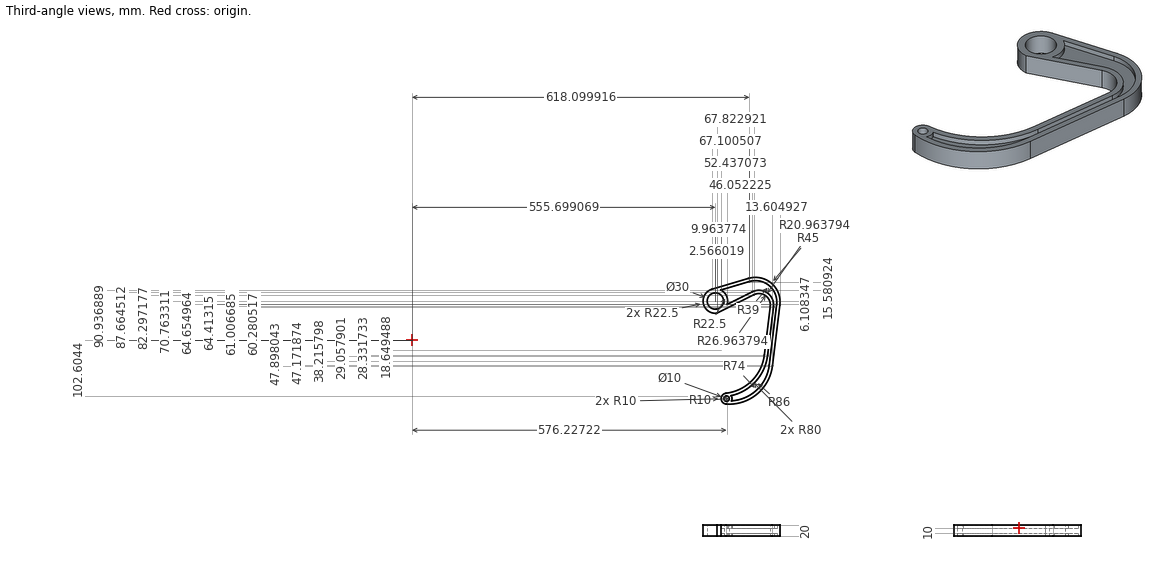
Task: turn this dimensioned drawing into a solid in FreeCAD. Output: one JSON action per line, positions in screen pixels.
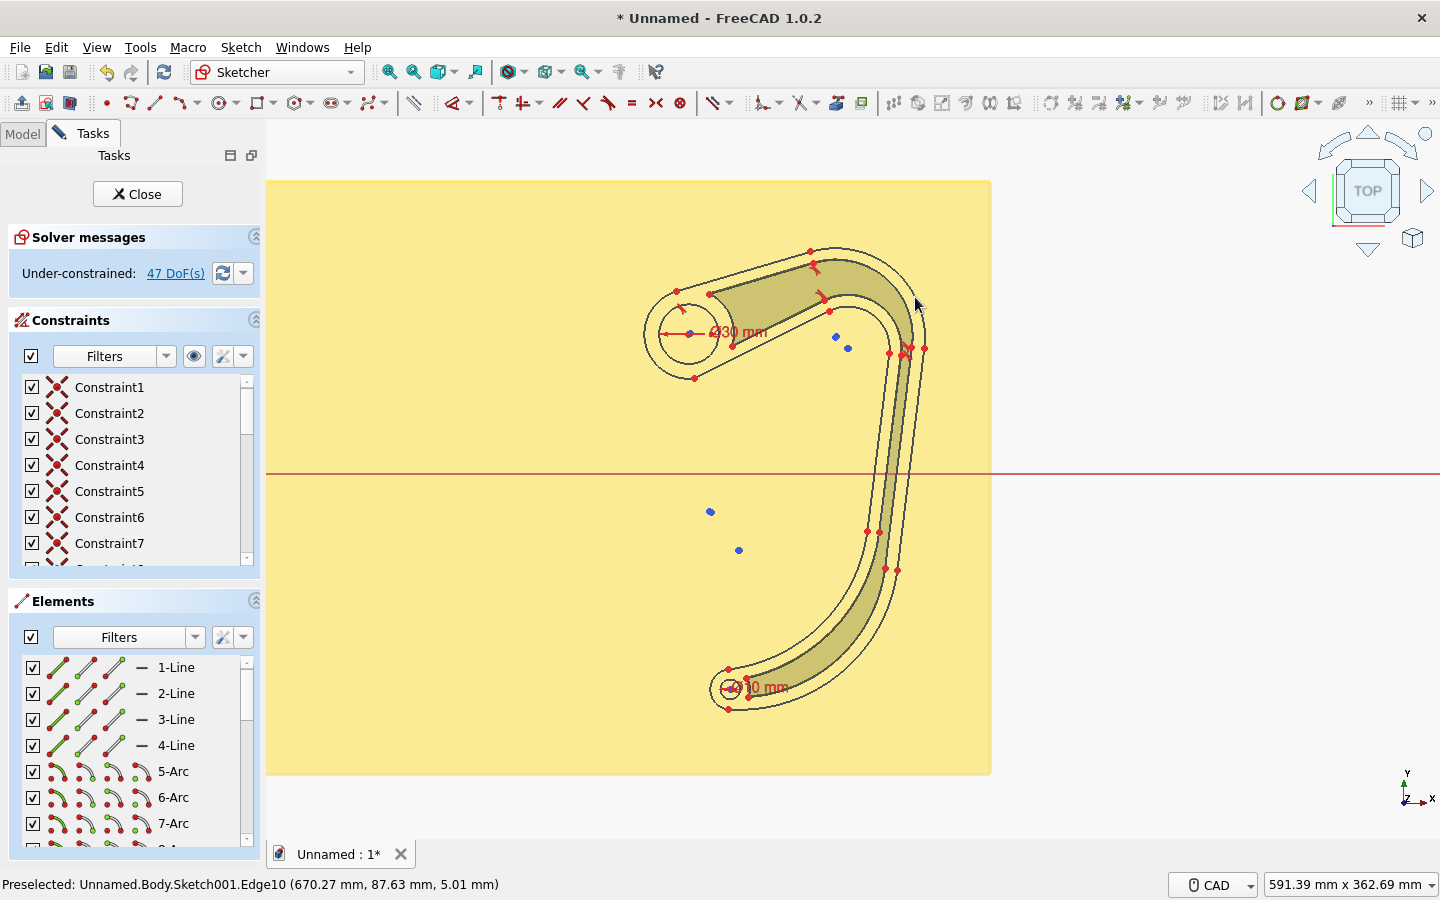
{"action": "left_click", "coordinate": [788, 650]}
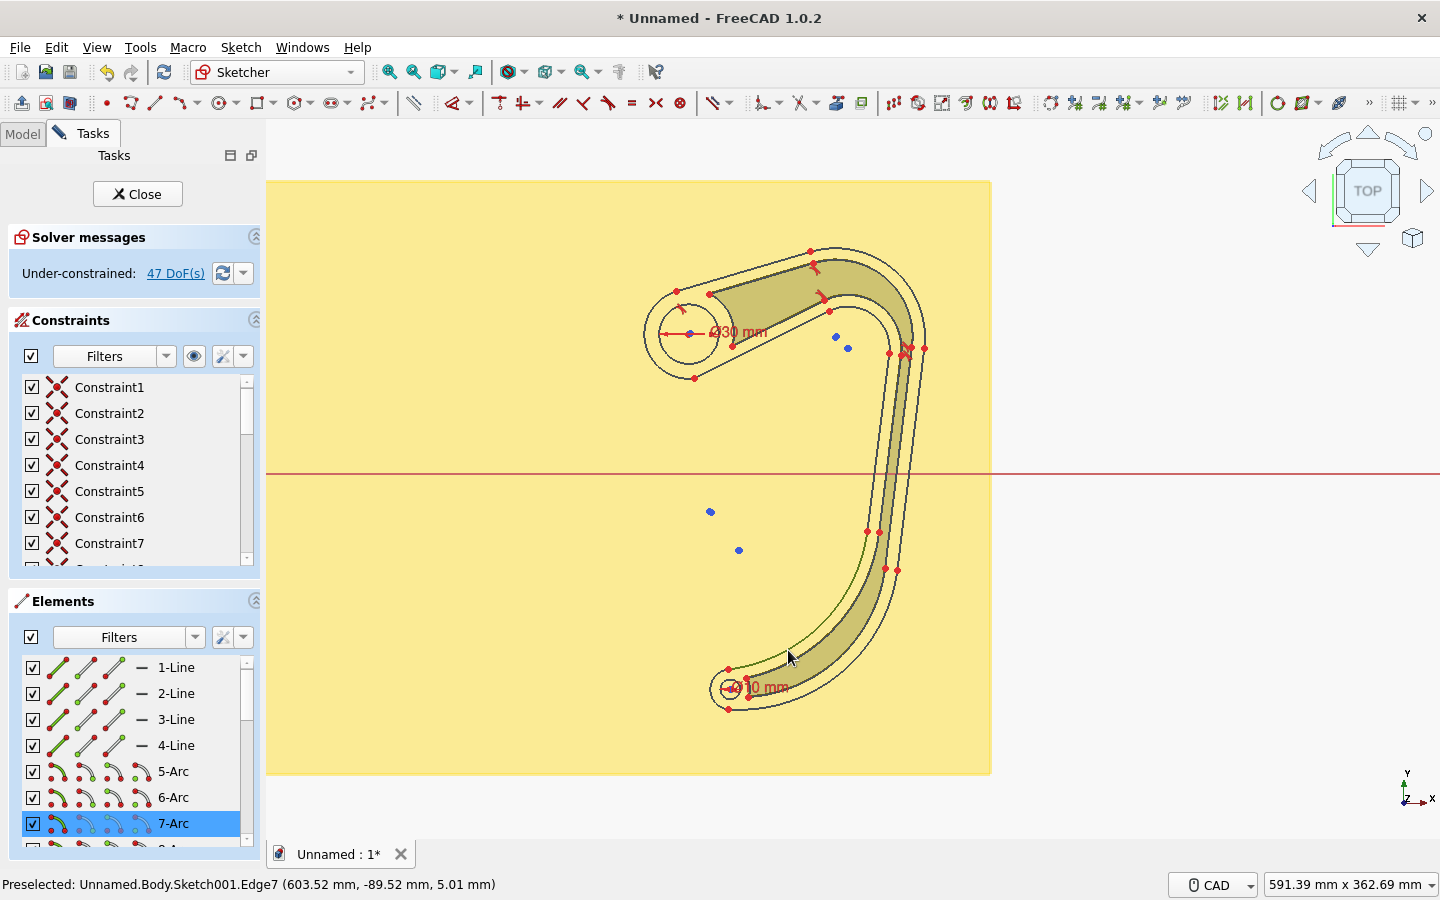
{"action": "scroll", "coordinate": [714, 678], "scroll_direction": "up", "scroll_amount": 2}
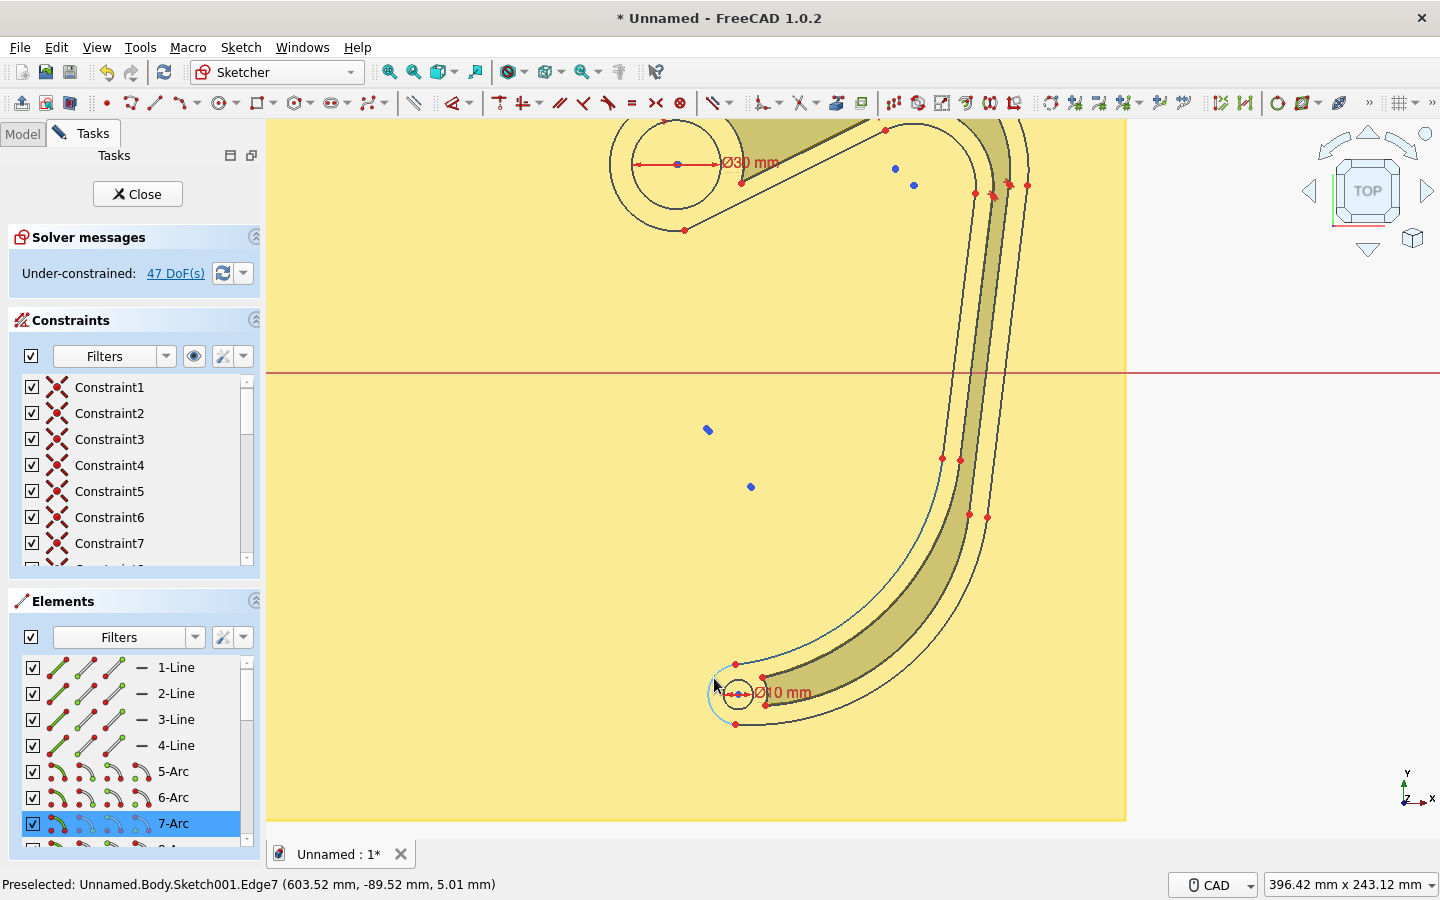
{"action": "left_click", "coordinate": [713, 678]}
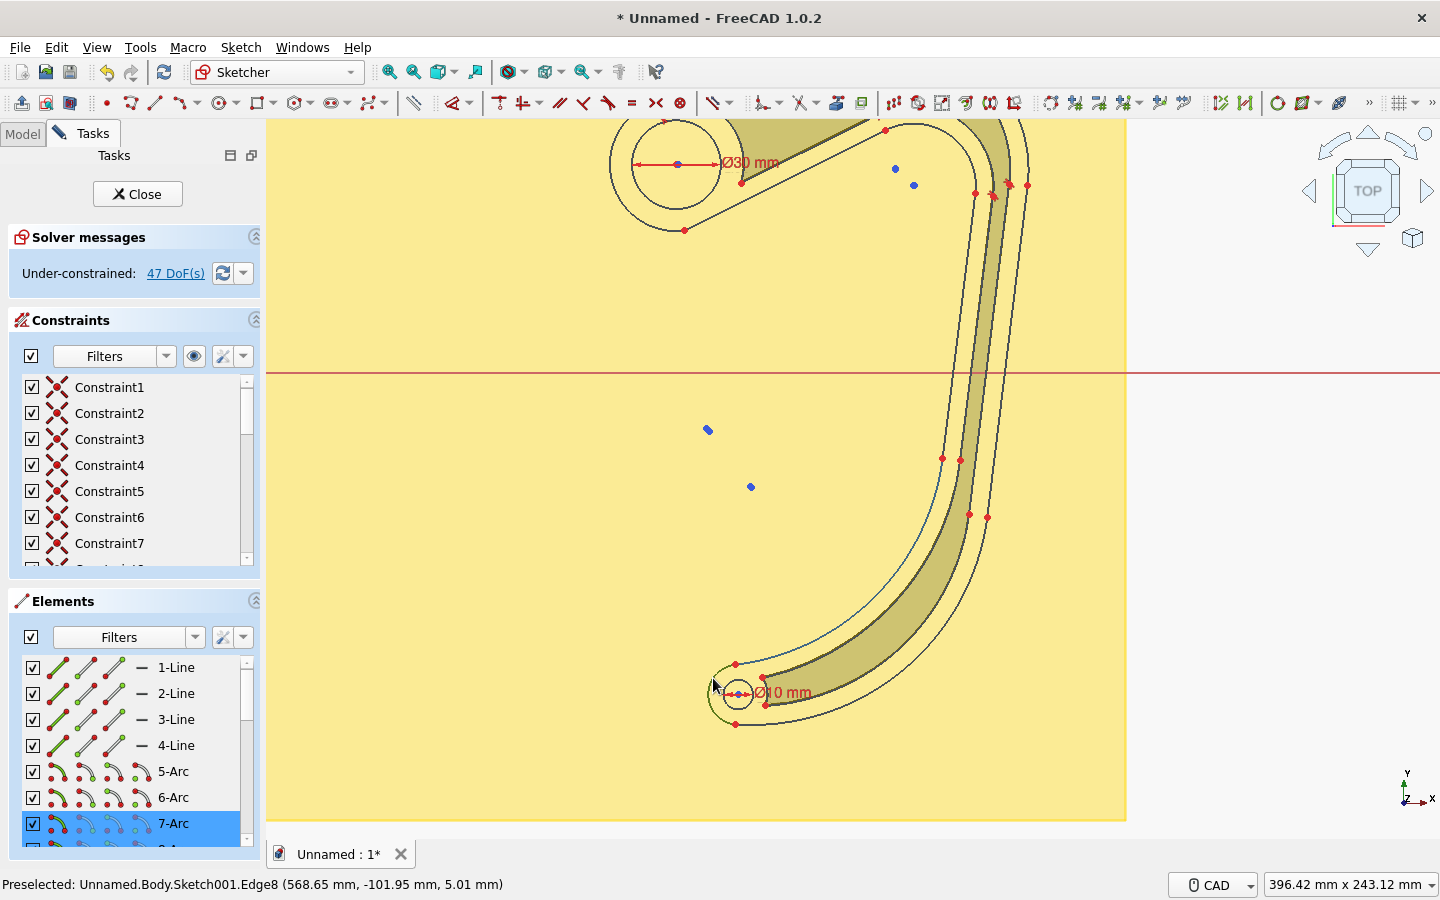
{"action": "left_click", "coordinate": [608, 104]}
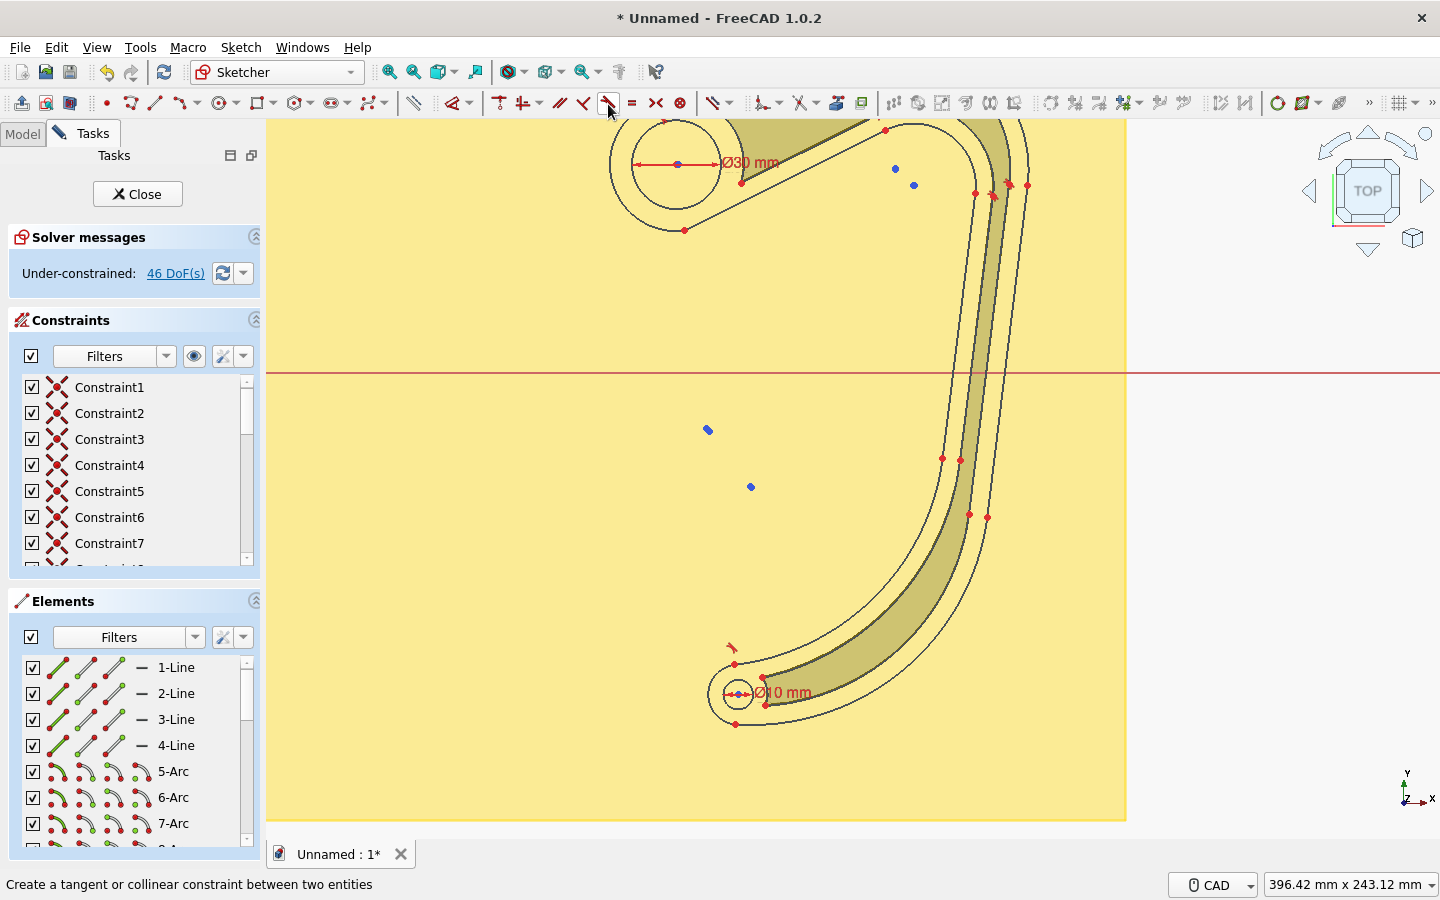
{"action": "left_click", "coordinate": [713, 678]}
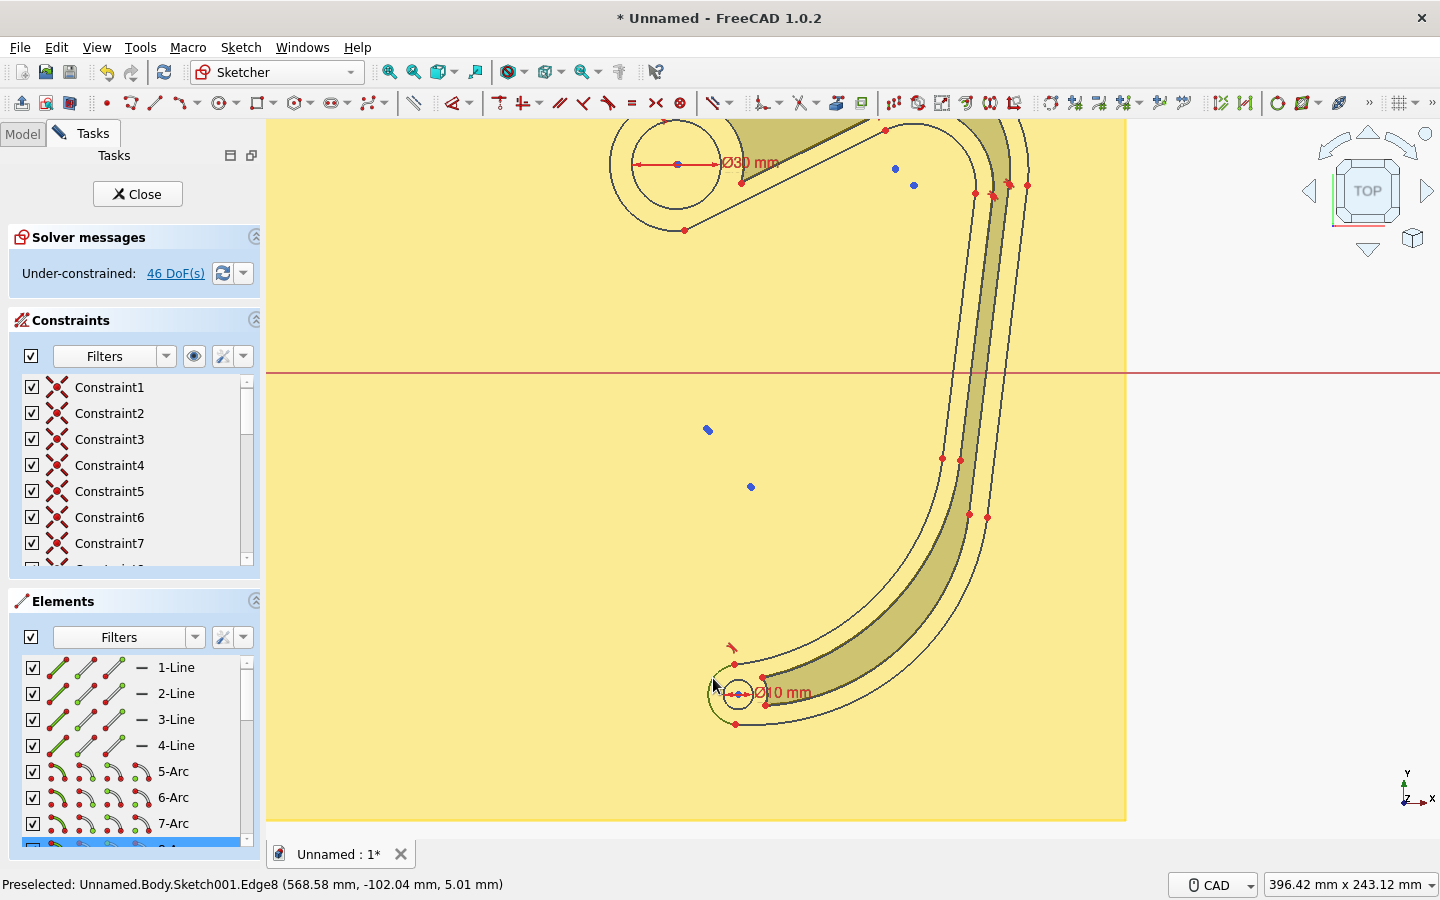
{"action": "left_click", "coordinate": [841, 707]}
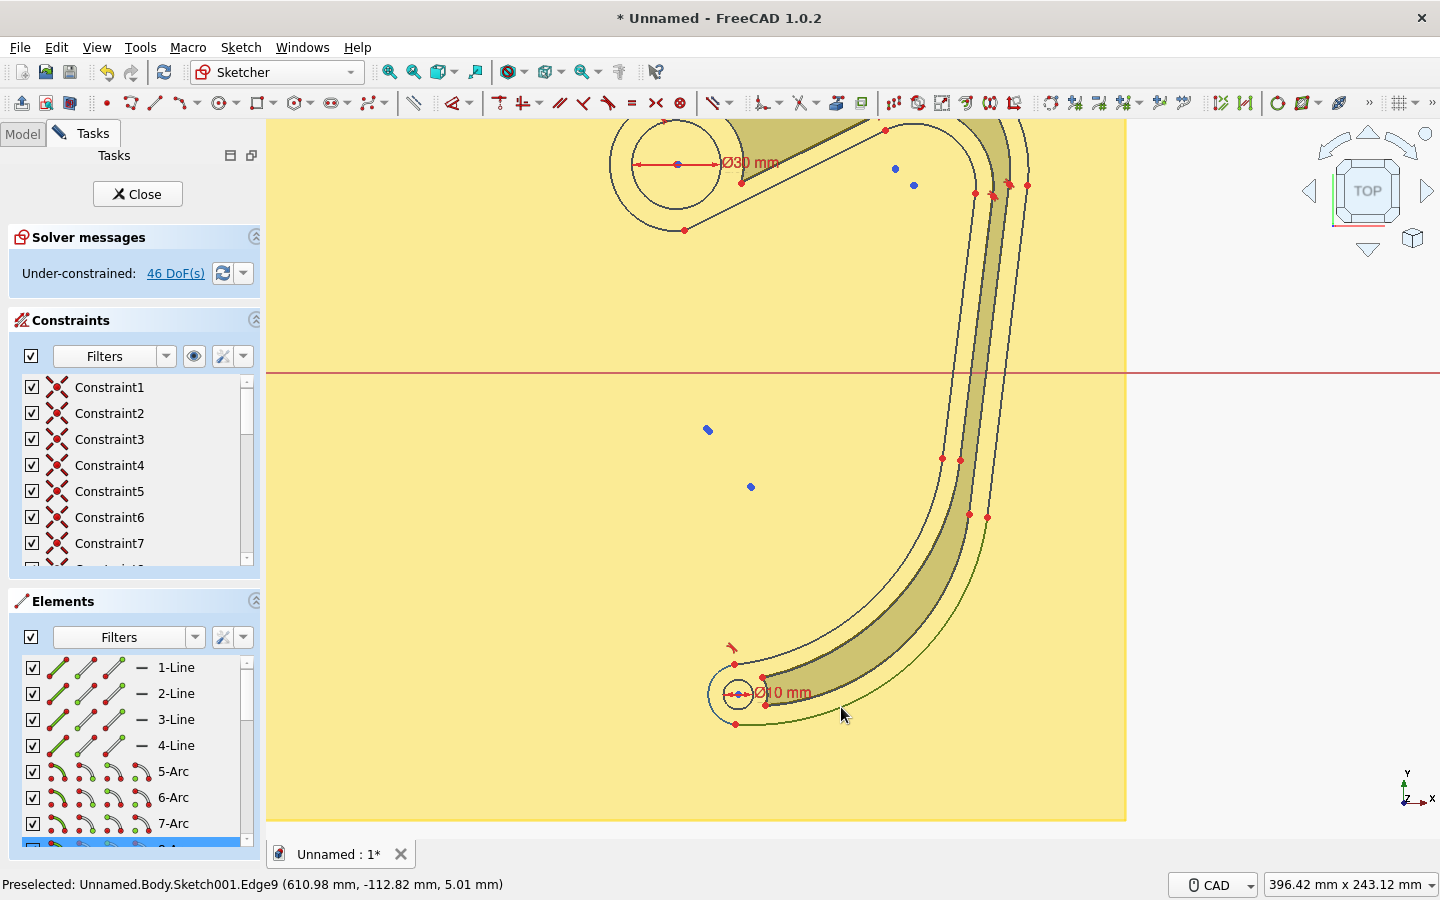
{"action": "left_click", "coordinate": [608, 104]}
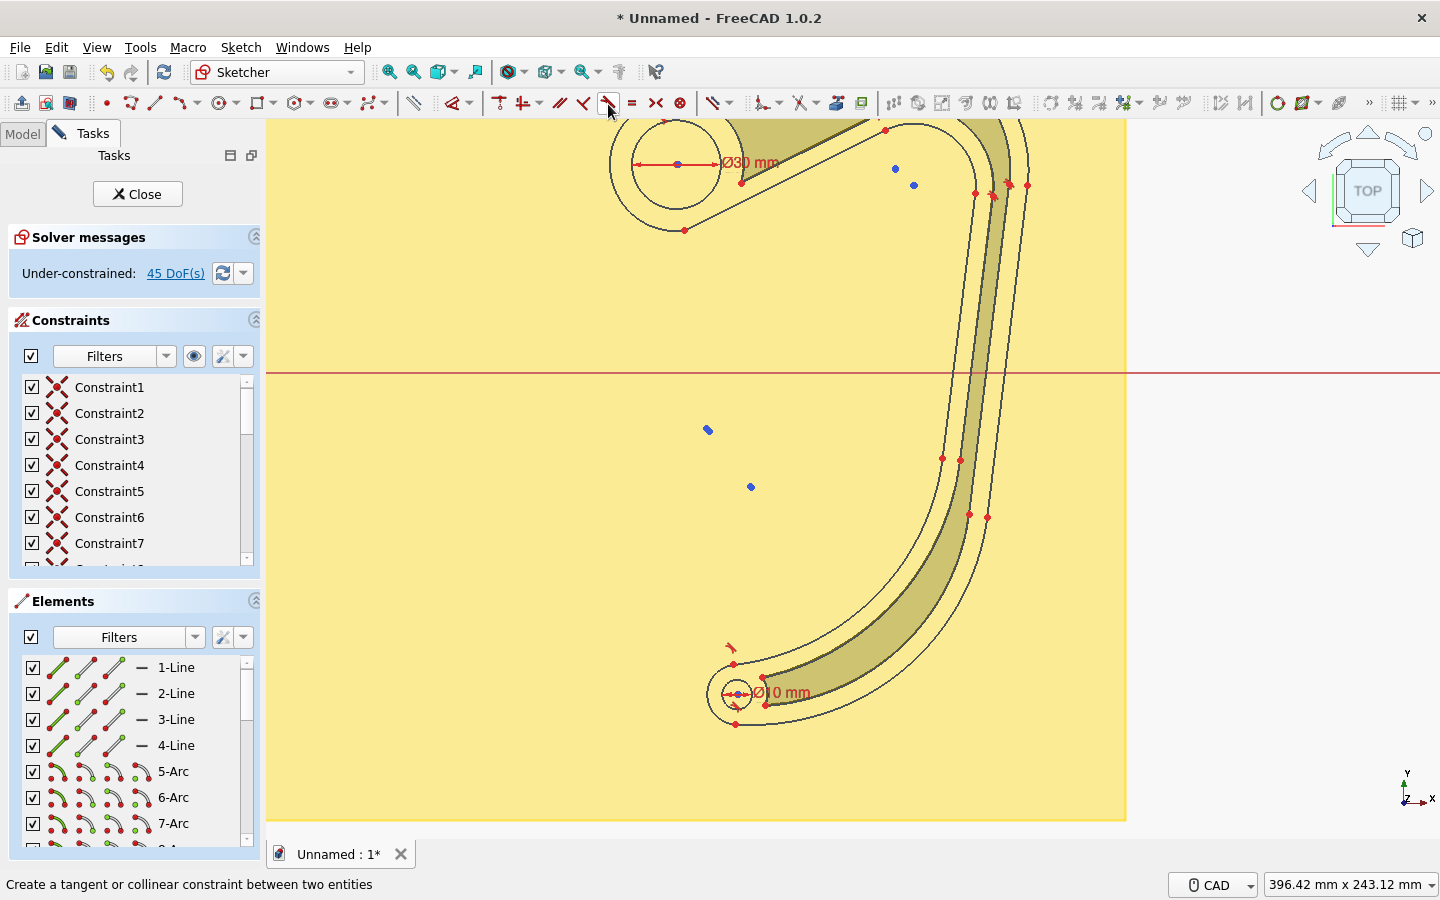
{"action": "scroll", "coordinate": [713, 677], "scroll_direction": "down", "scroll_amount": 2}